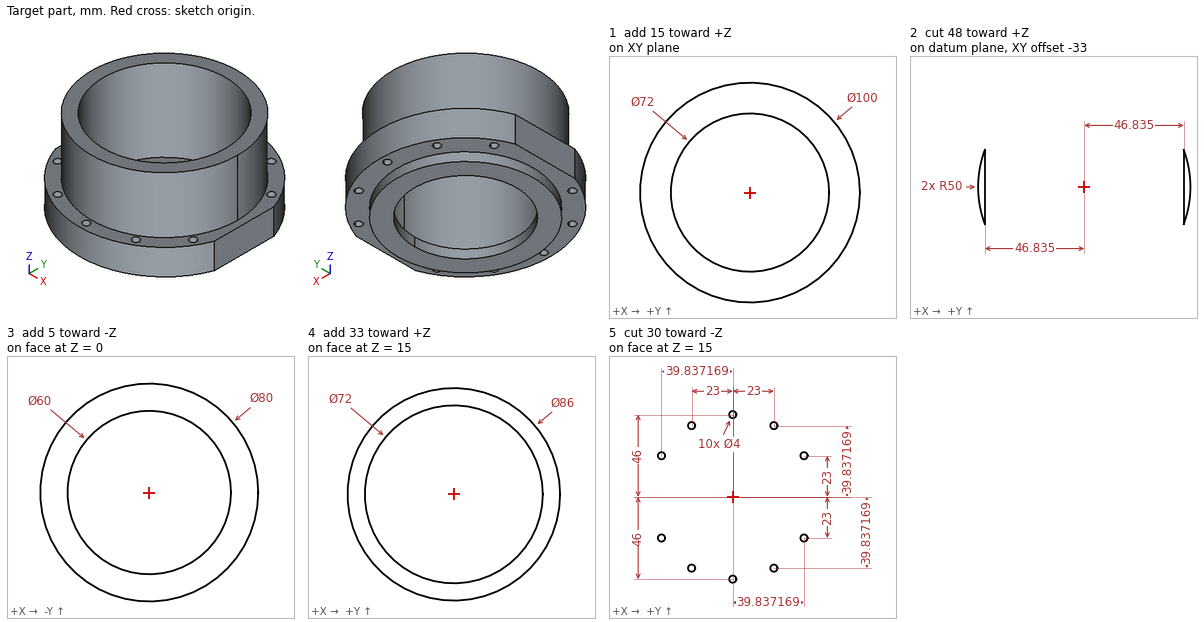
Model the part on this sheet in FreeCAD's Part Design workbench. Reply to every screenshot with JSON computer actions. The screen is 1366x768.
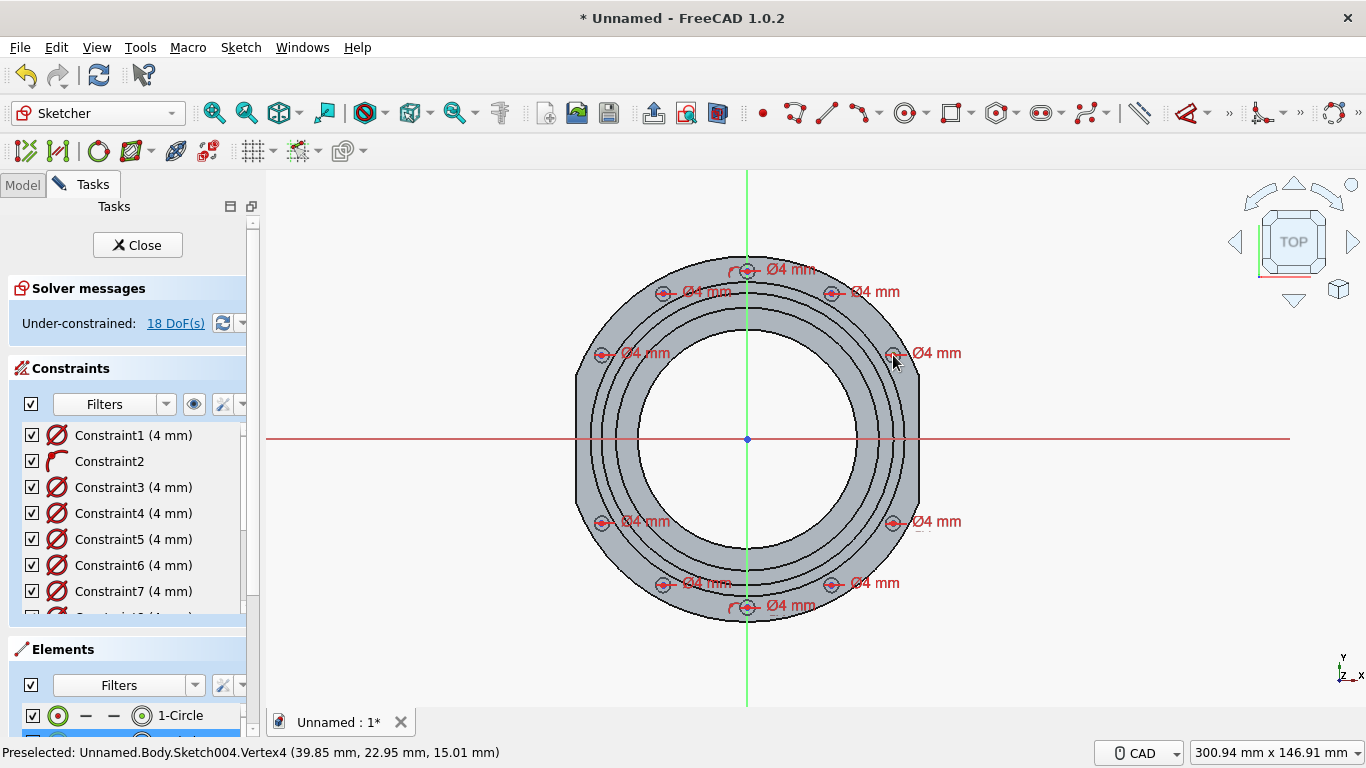
{"action": "key", "text": "v"}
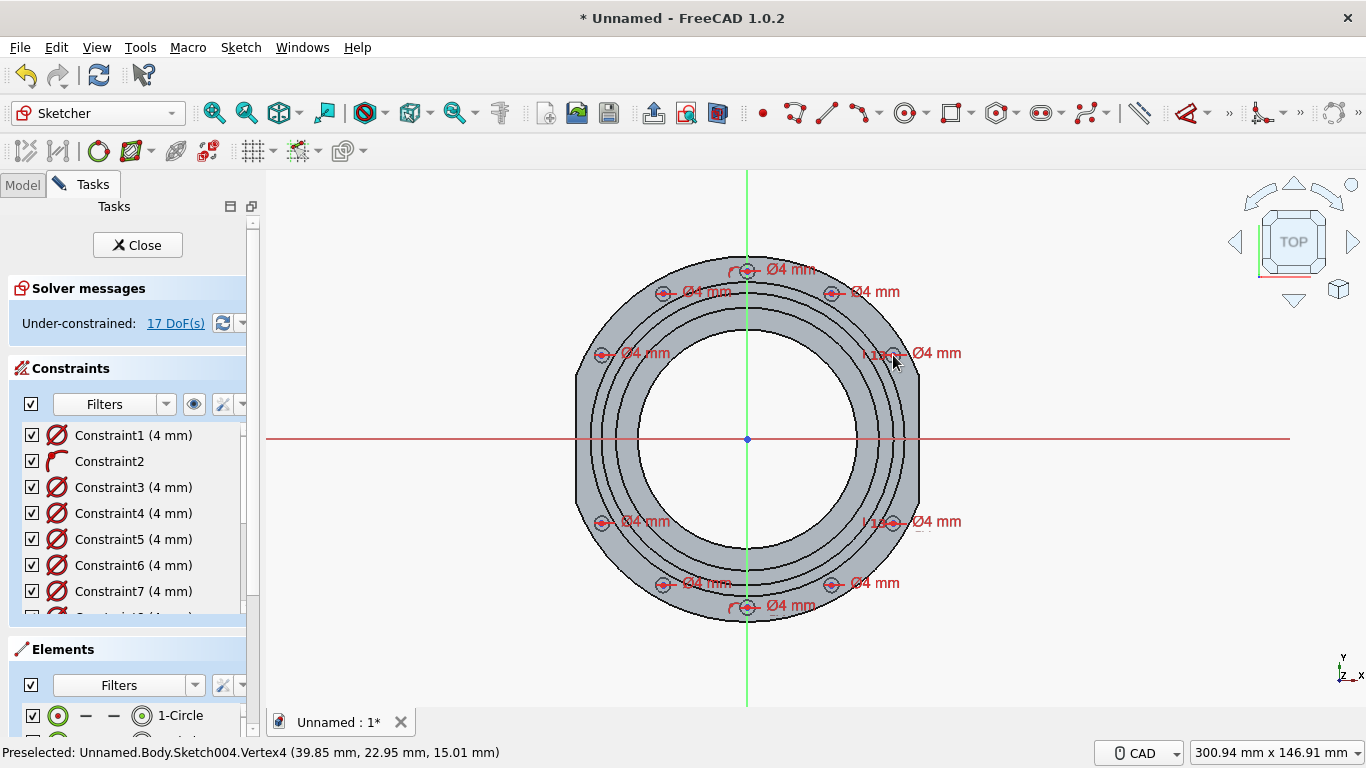
{"action": "left_click", "coordinate": [832, 294]}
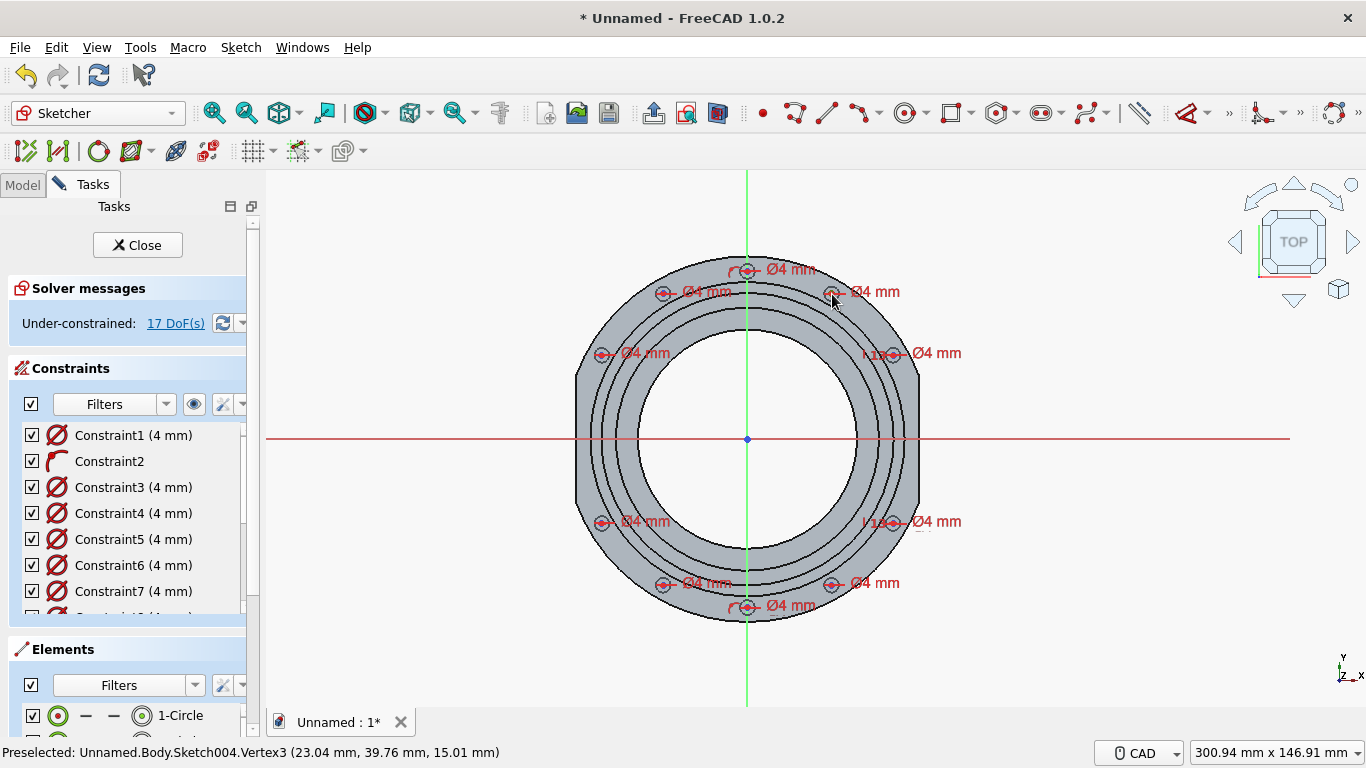
{"action": "left_click", "coordinate": [663, 294]}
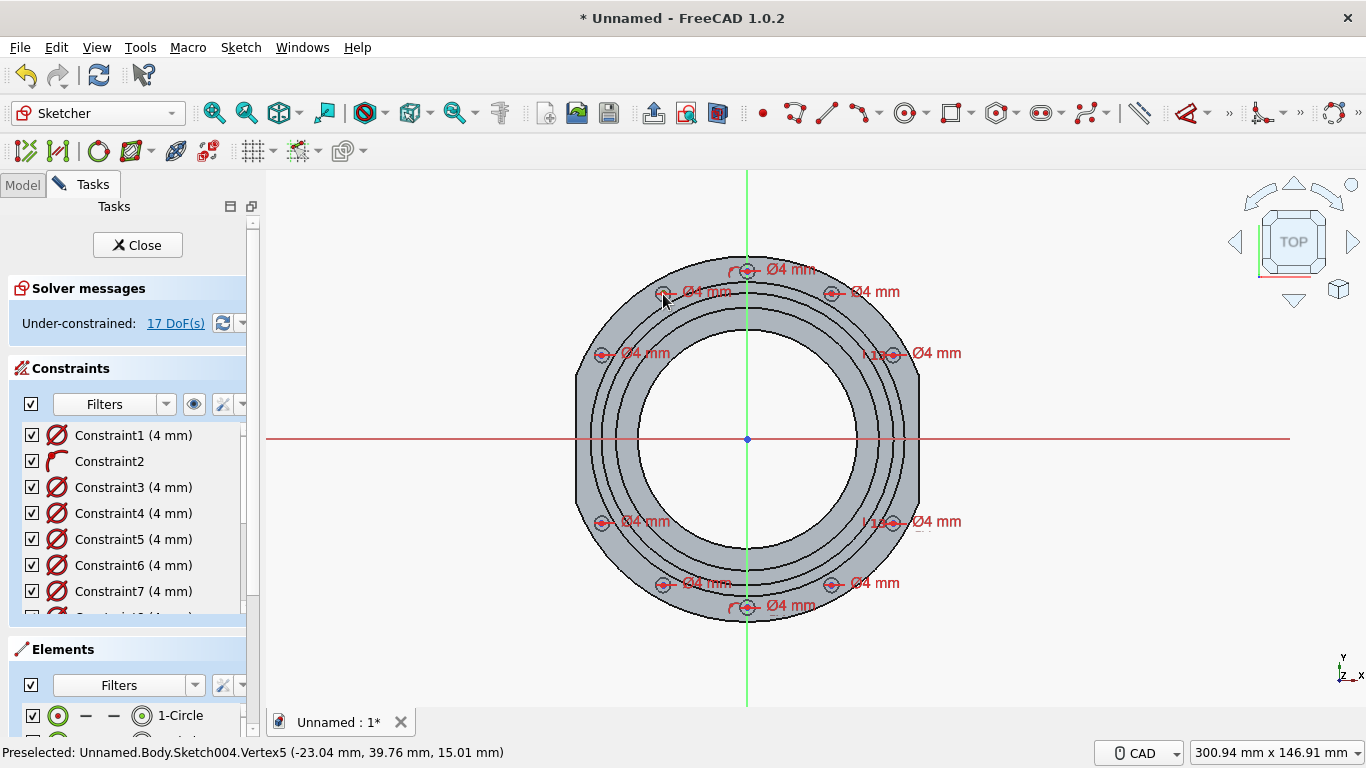
{"action": "key", "text": "h"}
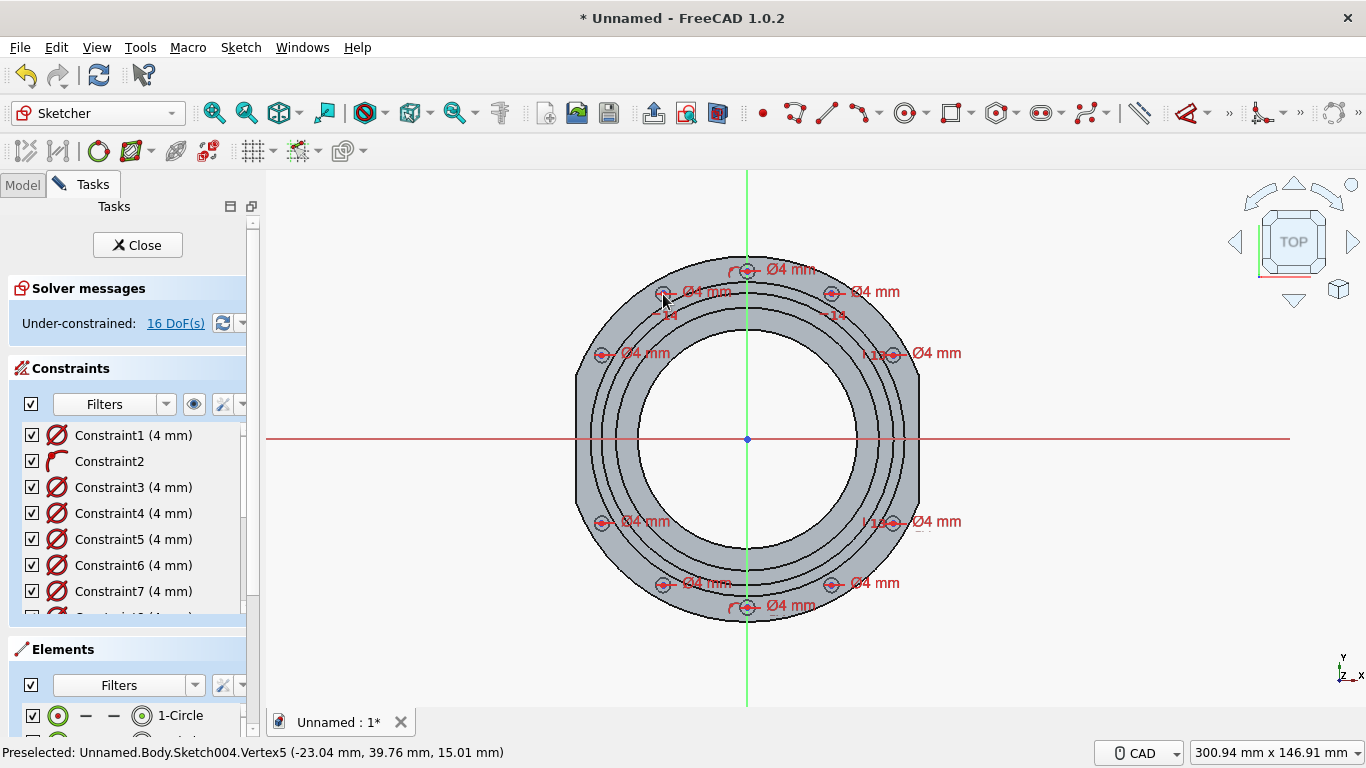
{"action": "left_click", "coordinate": [893, 355]}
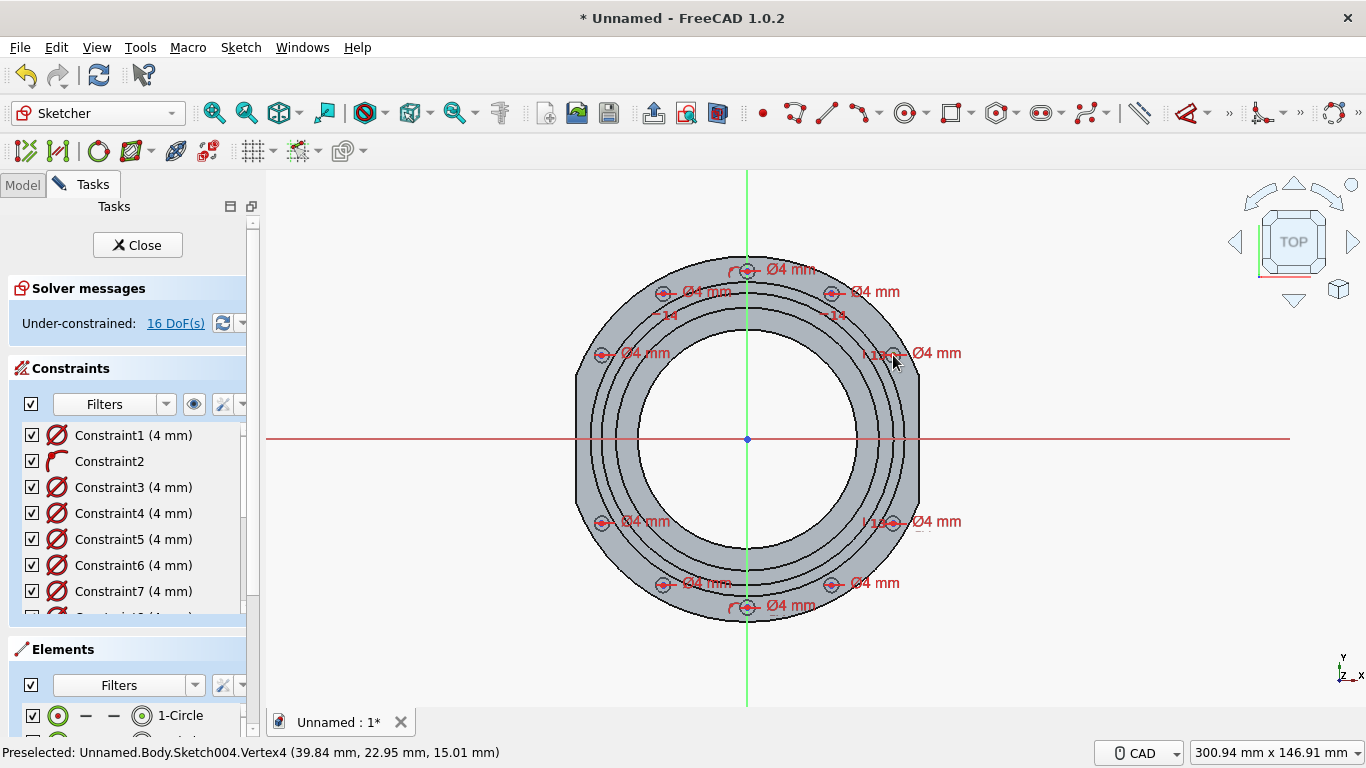
{"action": "left_click", "coordinate": [602, 355]}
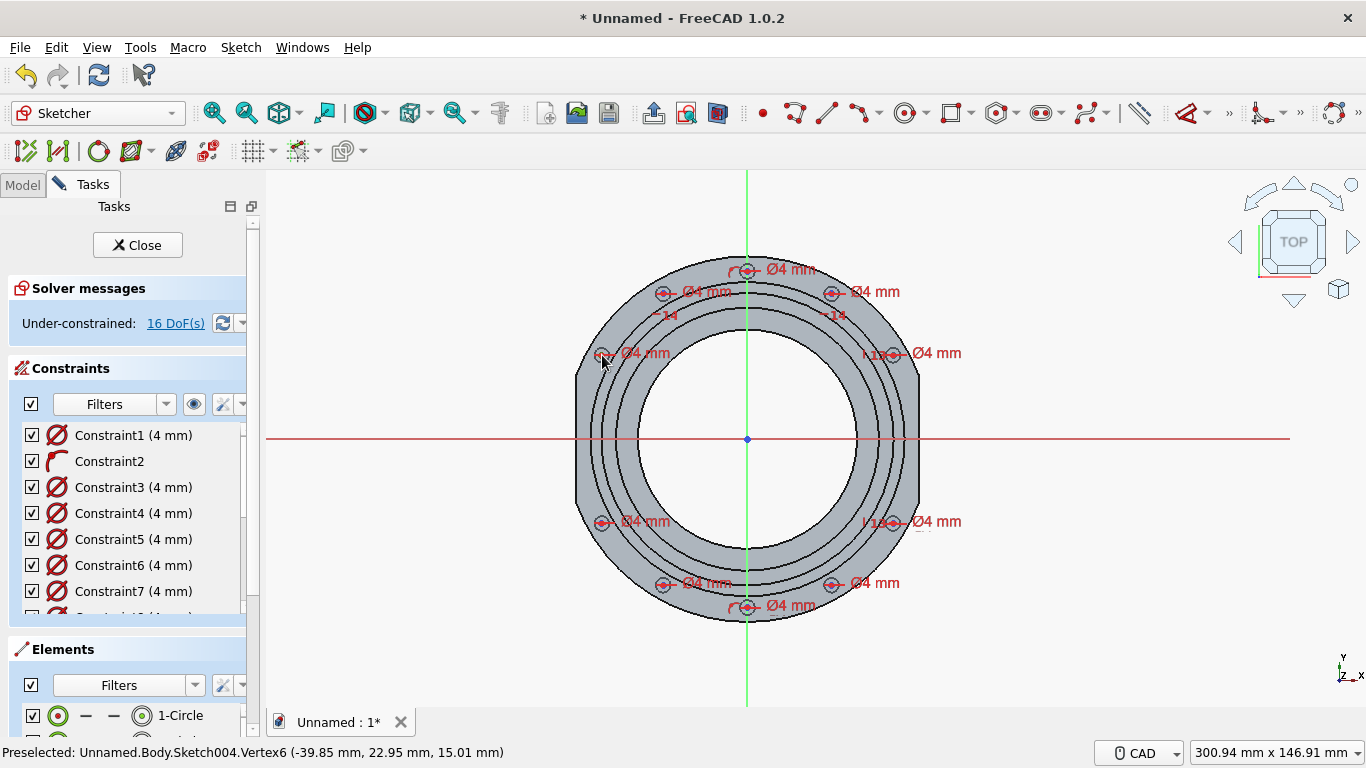
{"action": "key", "text": "h"}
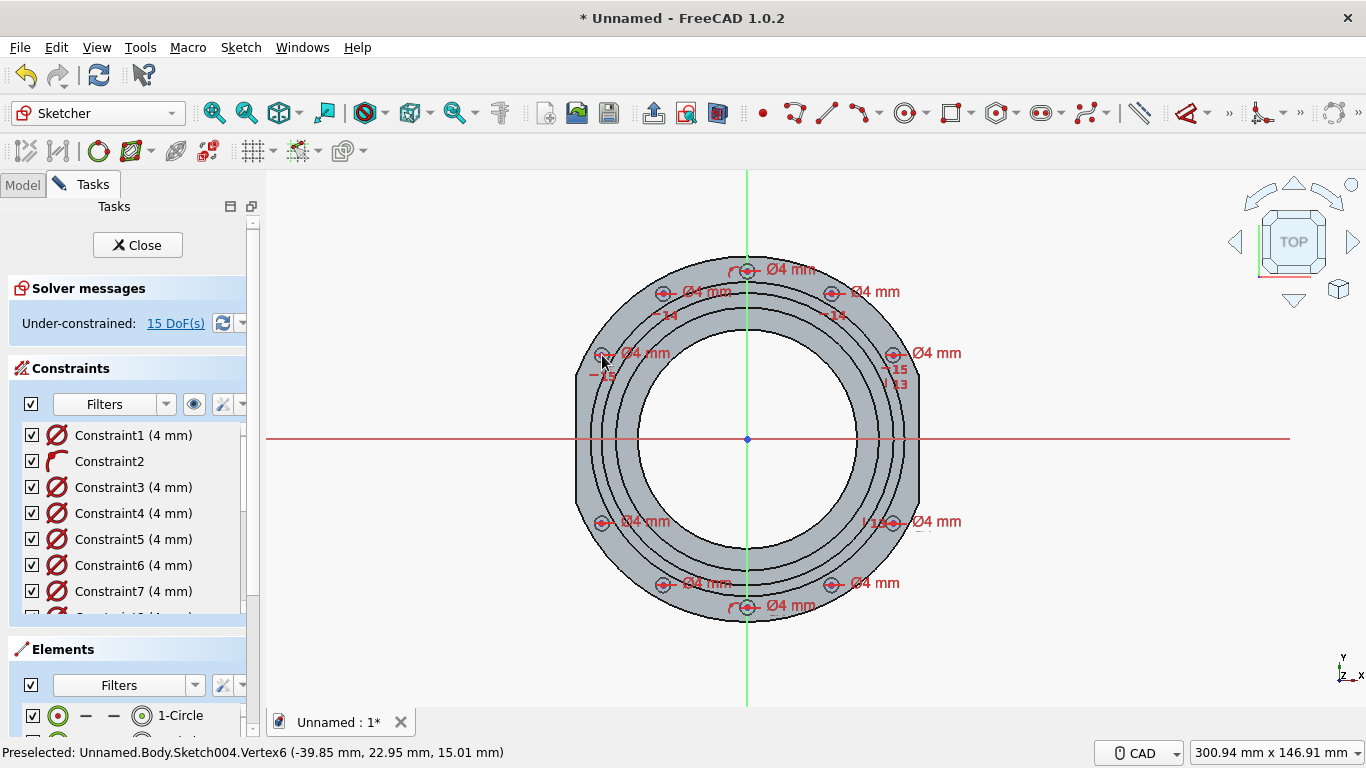
{"action": "left_click", "coordinate": [832, 294]}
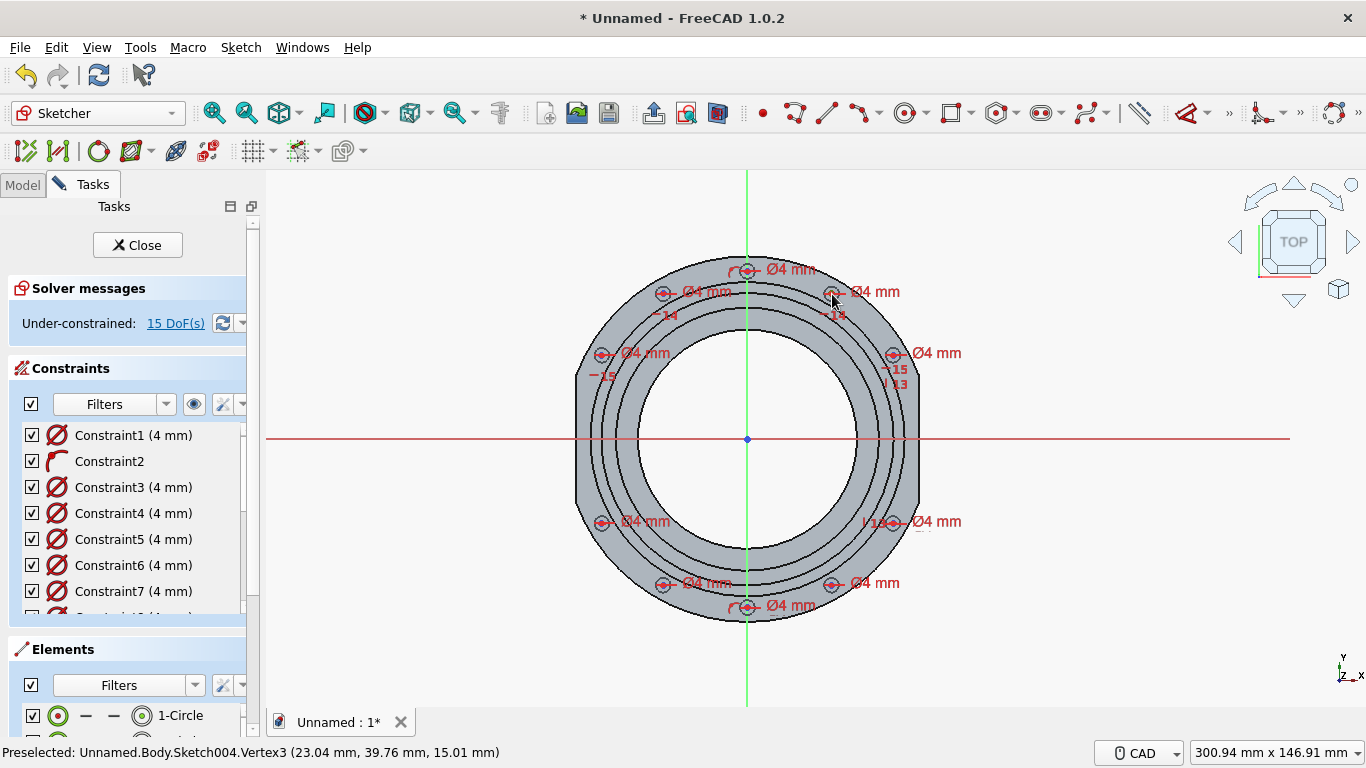
{"action": "left_click", "coordinate": [831, 585]}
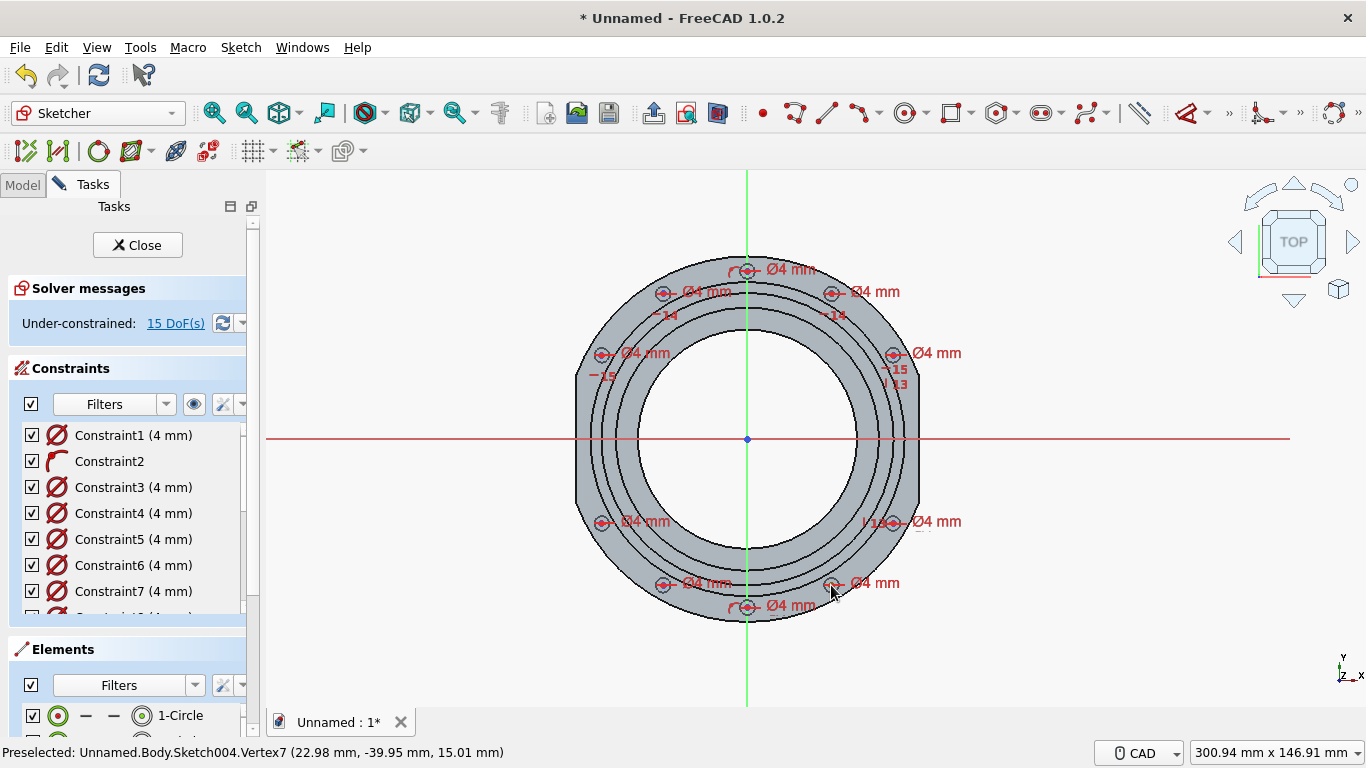
{"action": "key", "text": "v"}